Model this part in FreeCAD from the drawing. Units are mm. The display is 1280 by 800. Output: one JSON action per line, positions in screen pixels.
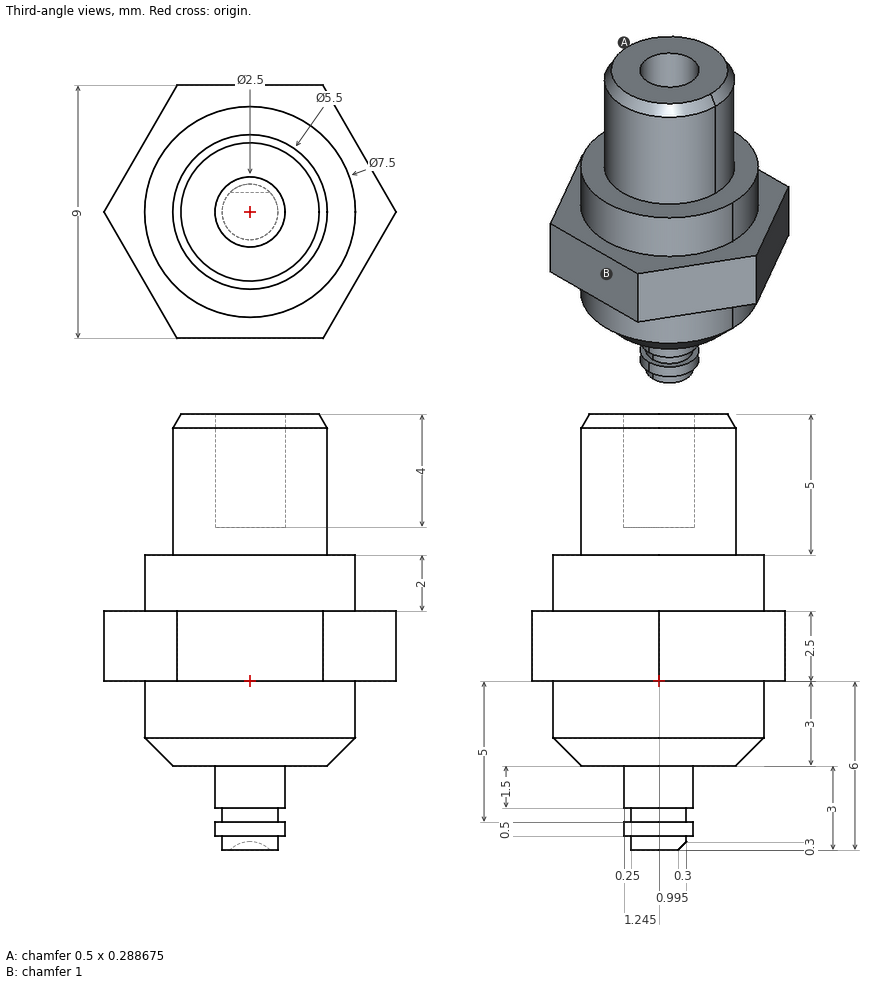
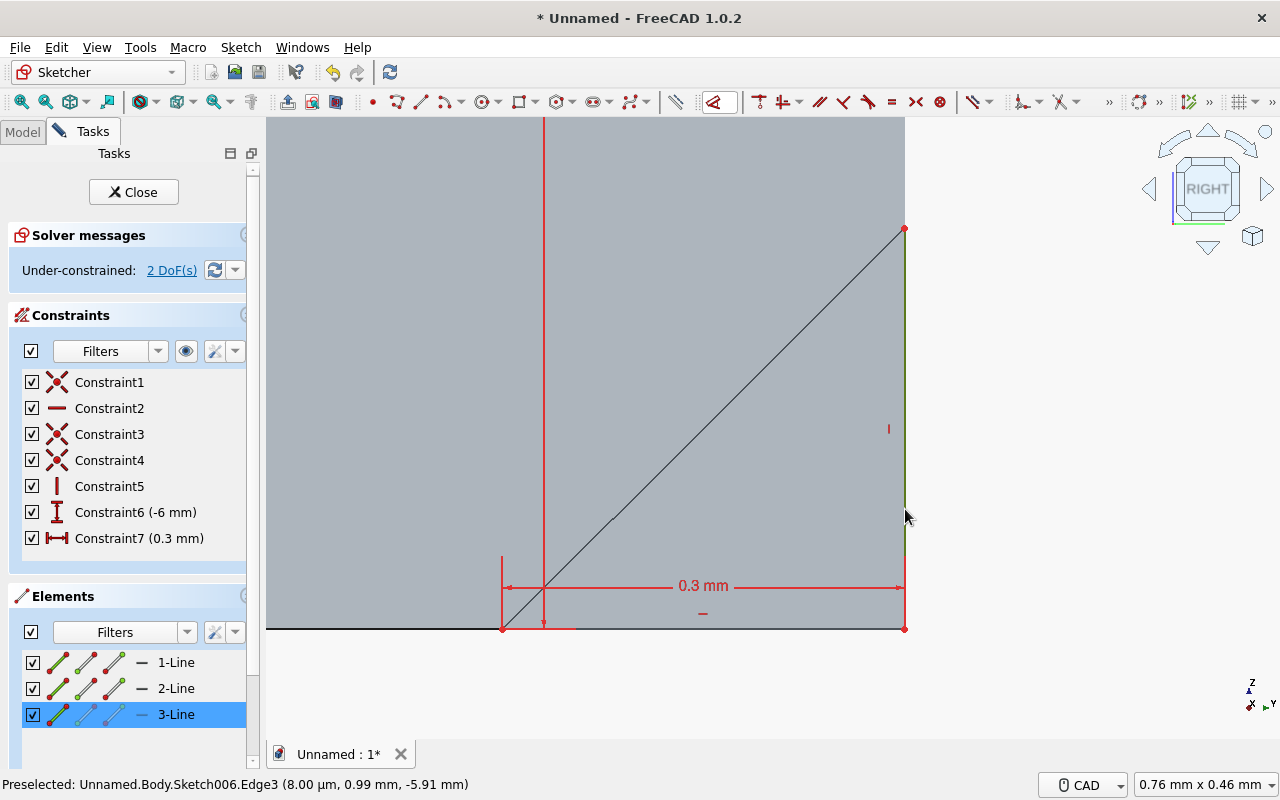
{"action": "key", "text": "i"}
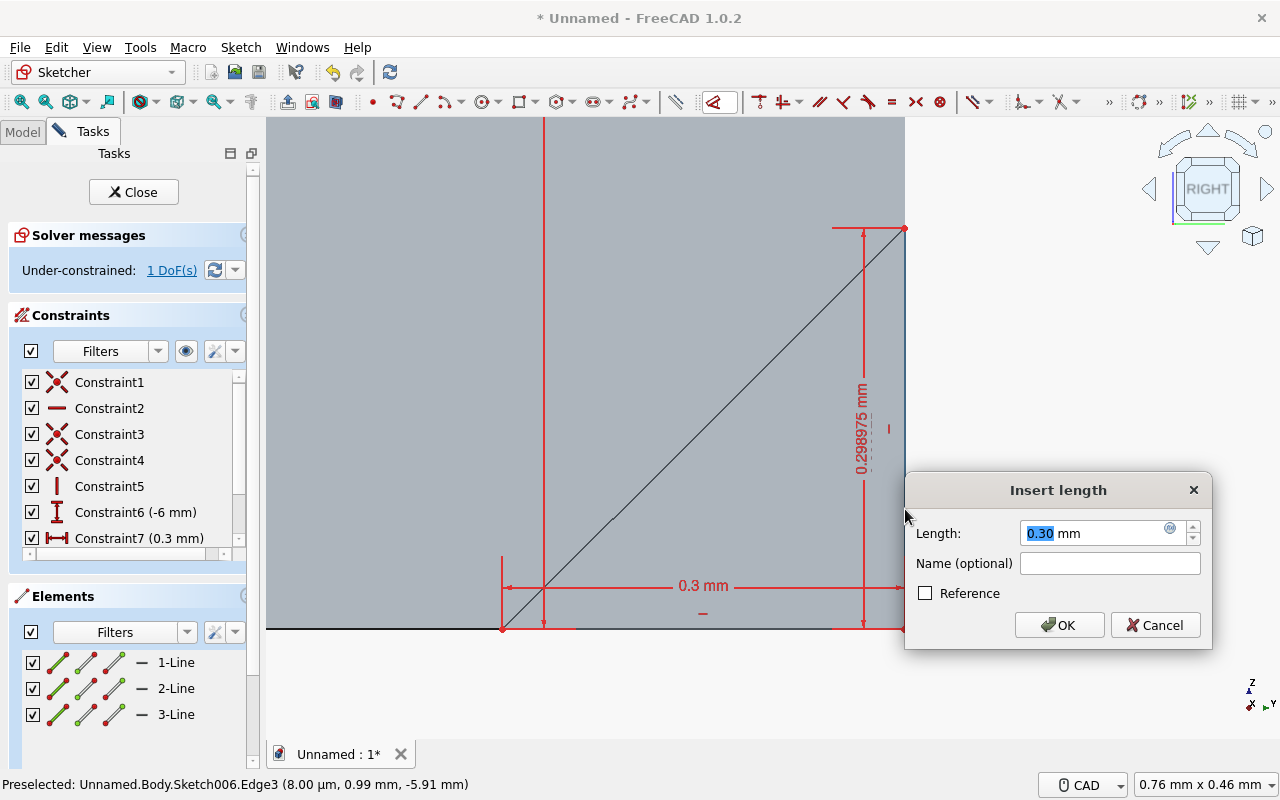
{"action": "type", "text": "0.3"}
{"action": "key", "text": "Return"}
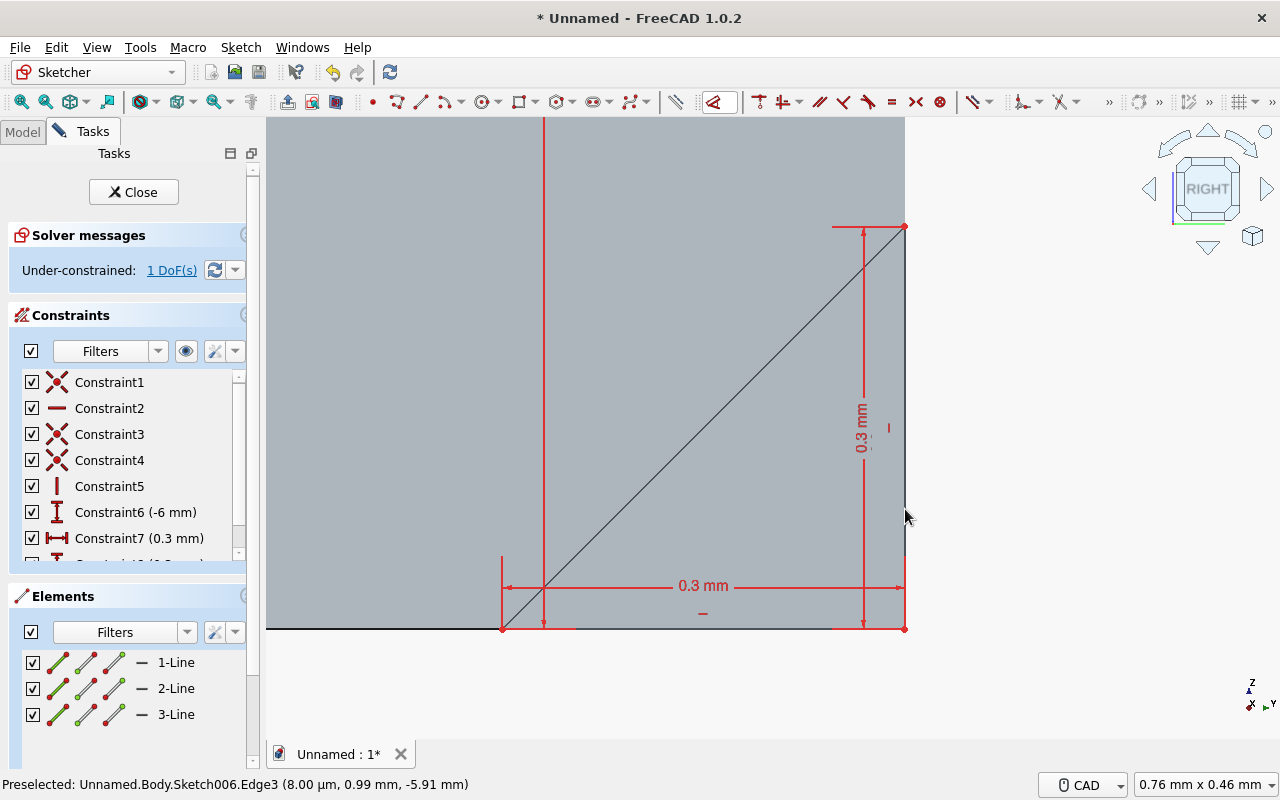
{"action": "left_click", "coordinate": [905, 227]}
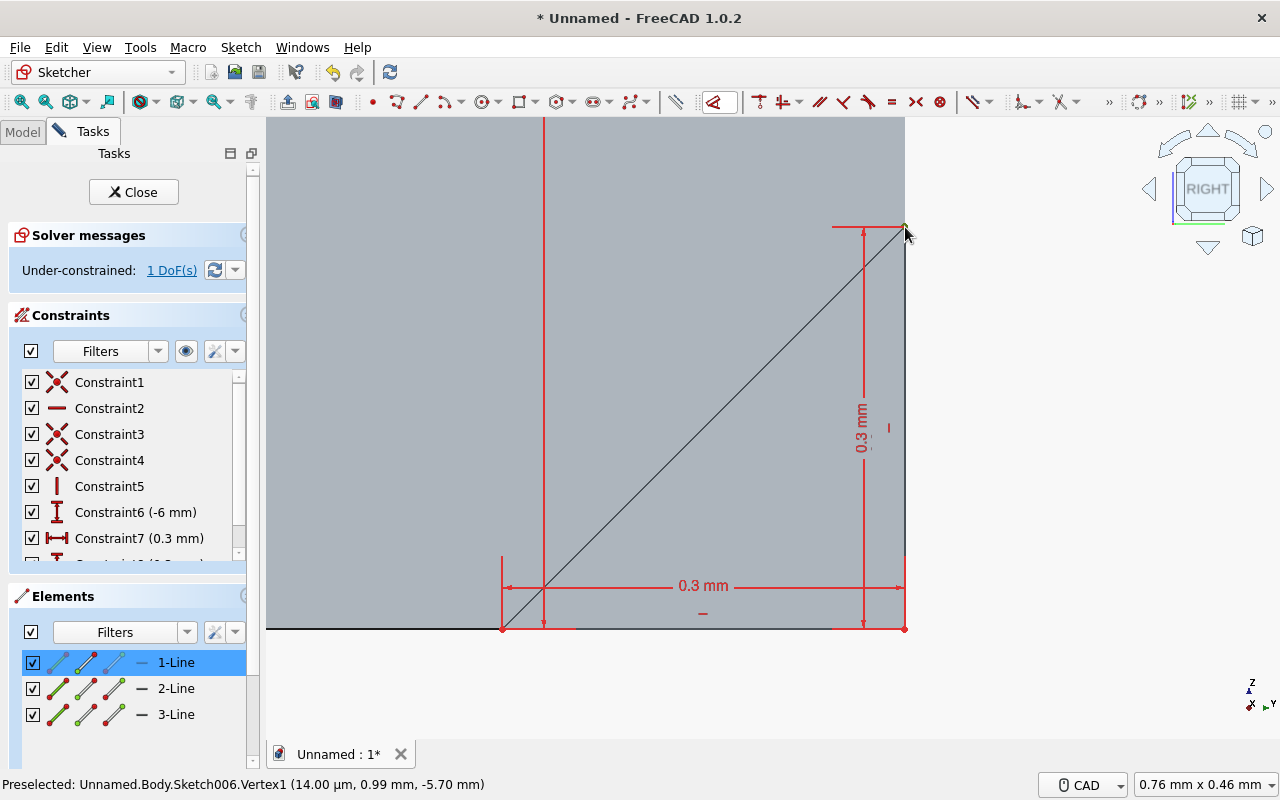
{"action": "key", "text": "l"}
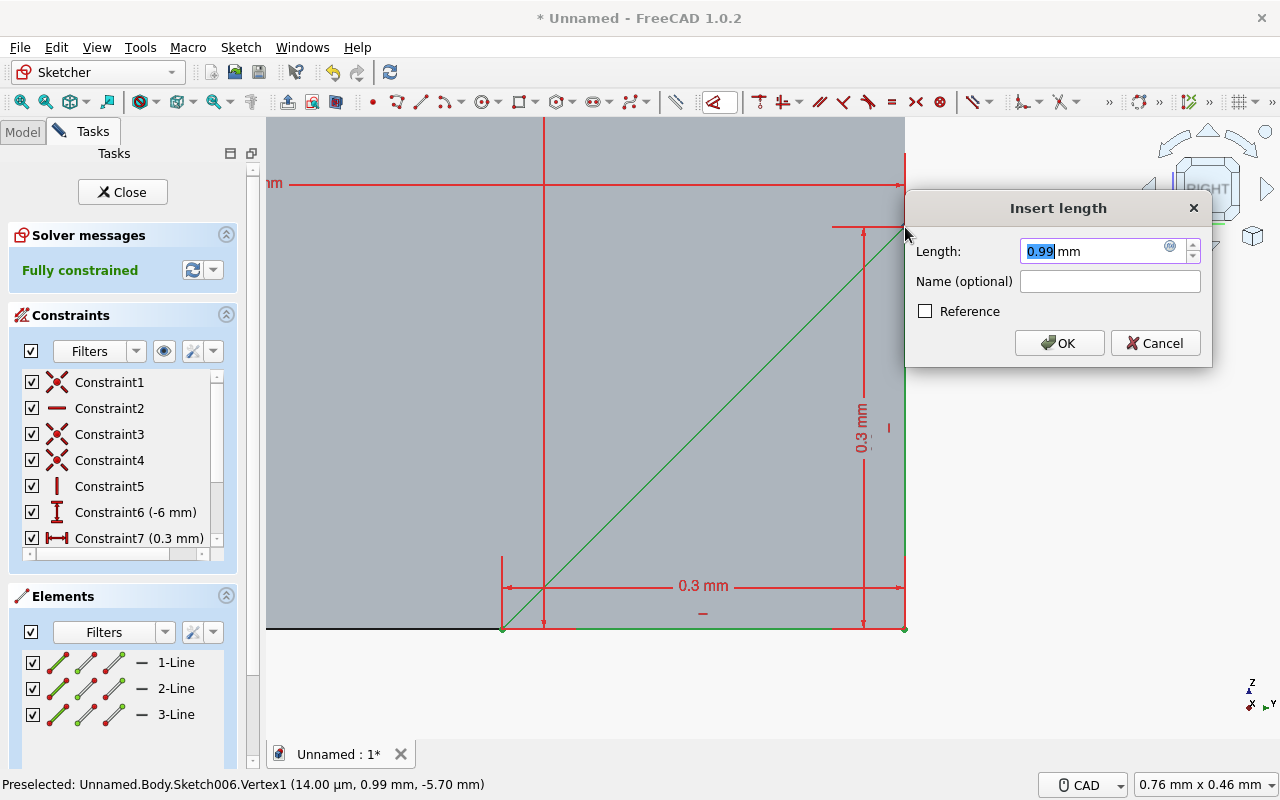
{"action": "type", "text": "0.995"}
{"action": "key", "text": "Return"}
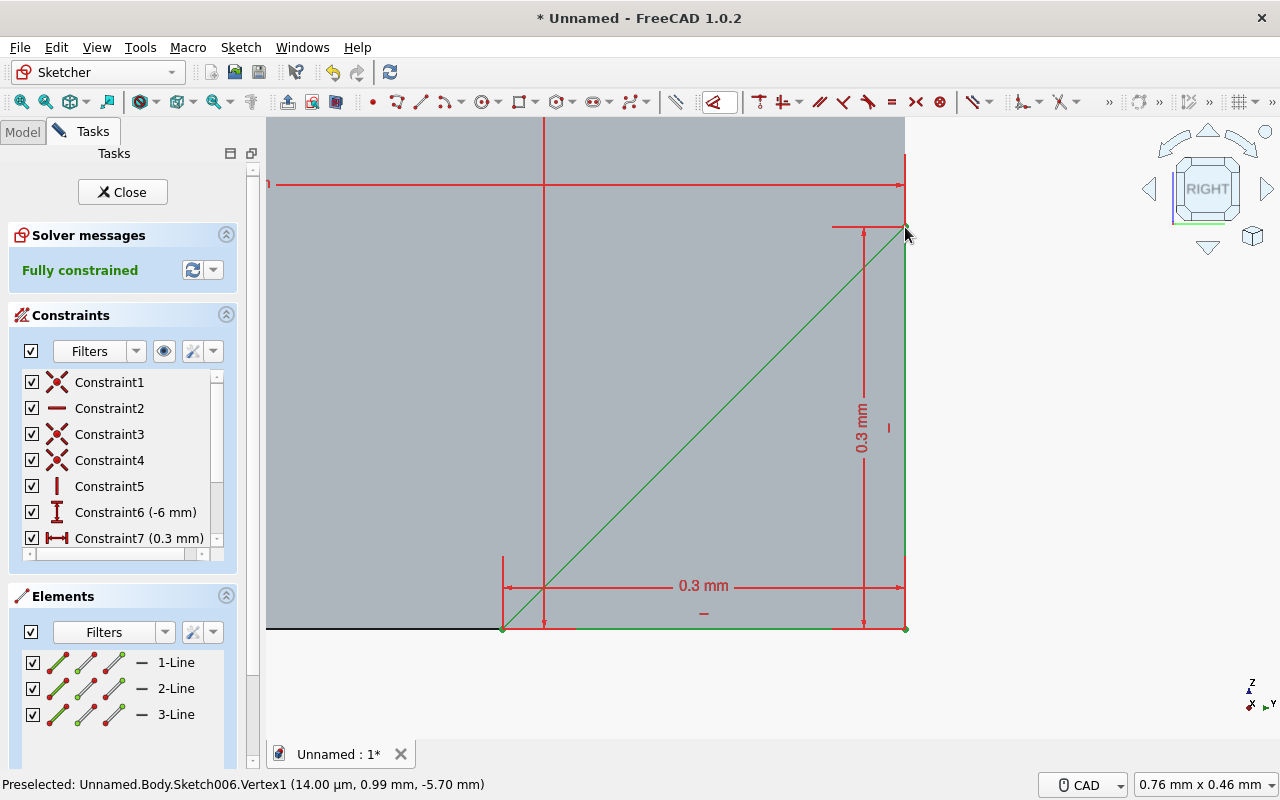
{"action": "left_click", "coordinate": [123, 192]}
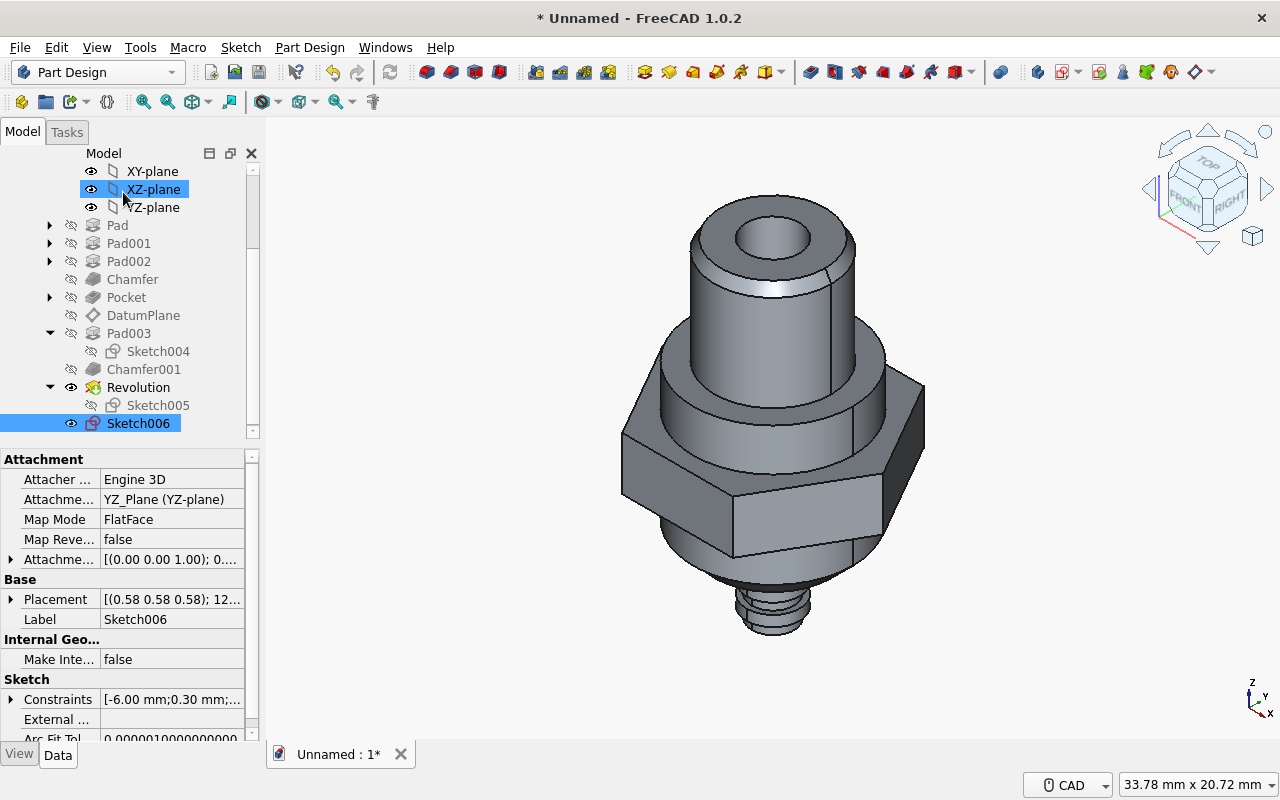
{"action": "left_click", "coordinate": [812, 72]}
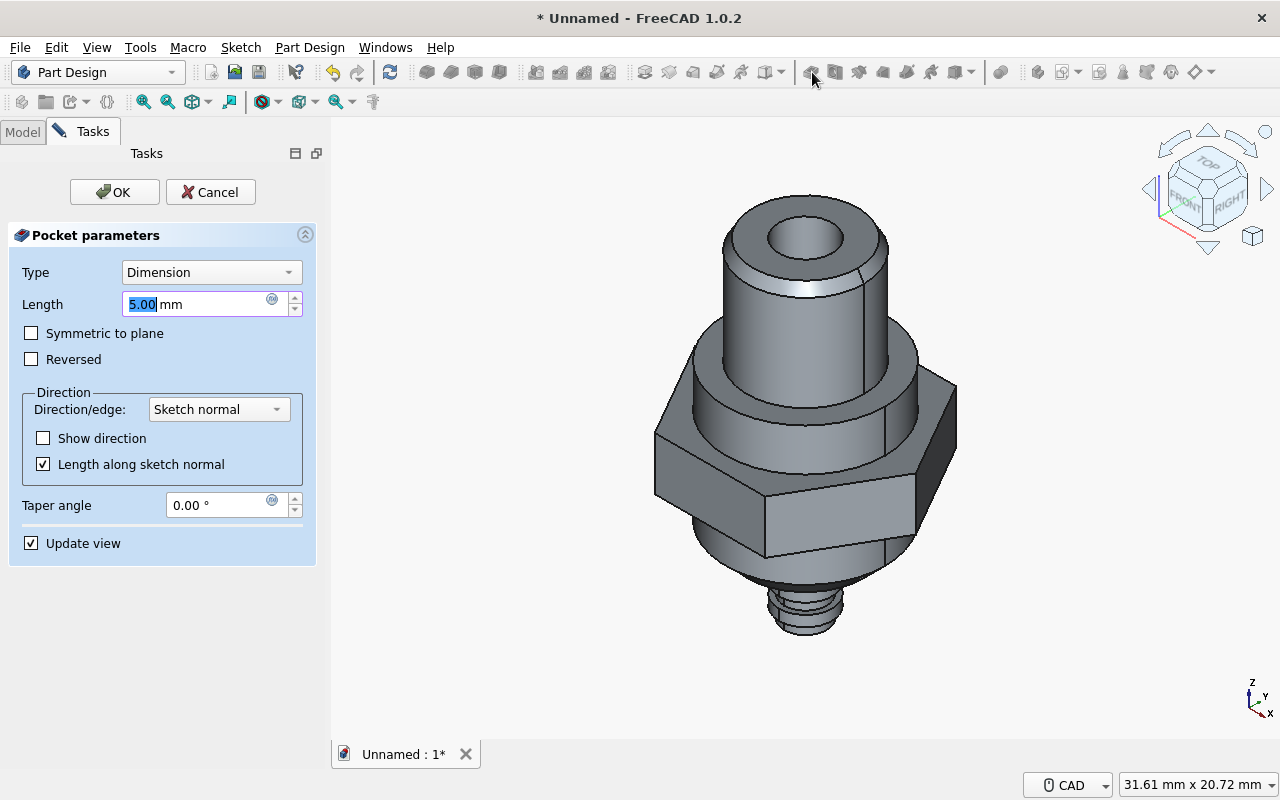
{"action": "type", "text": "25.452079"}
{"action": "key", "text": "Tab"}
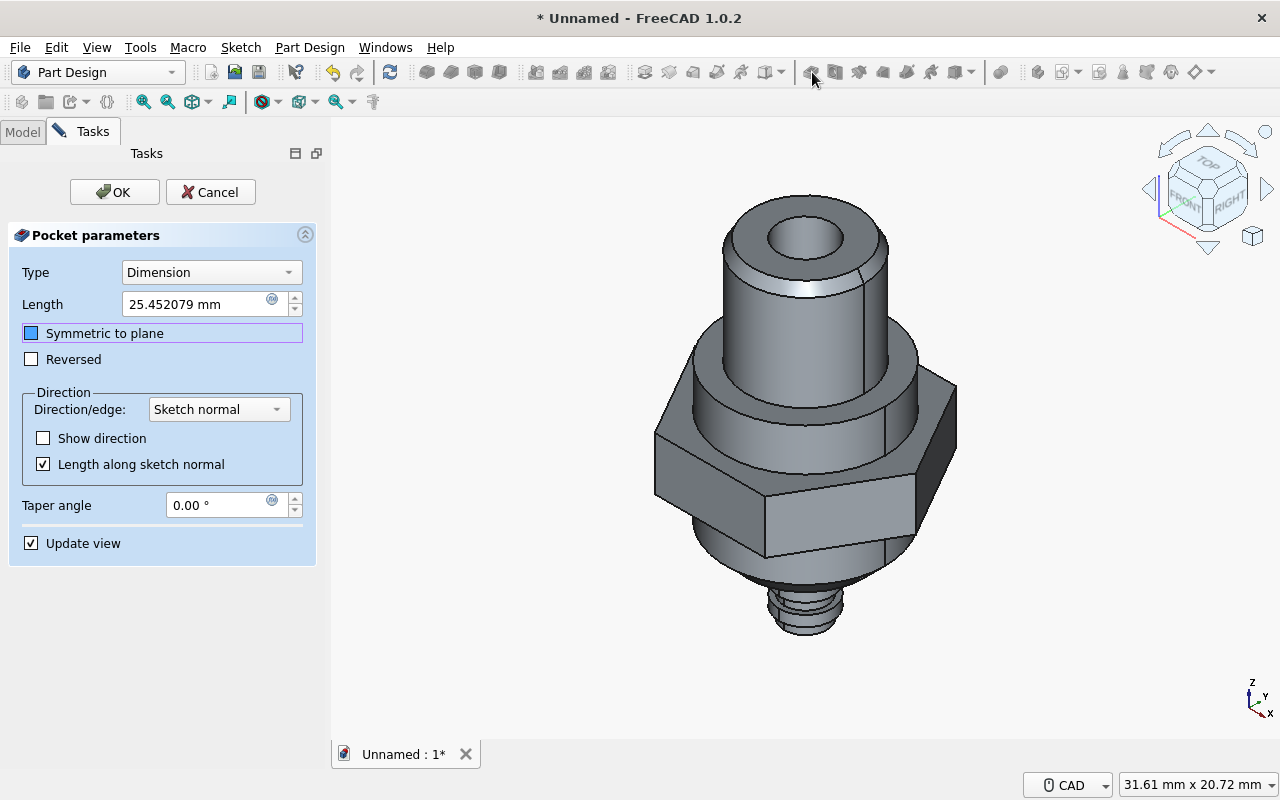
{"action": "left_click", "coordinate": [30, 333]}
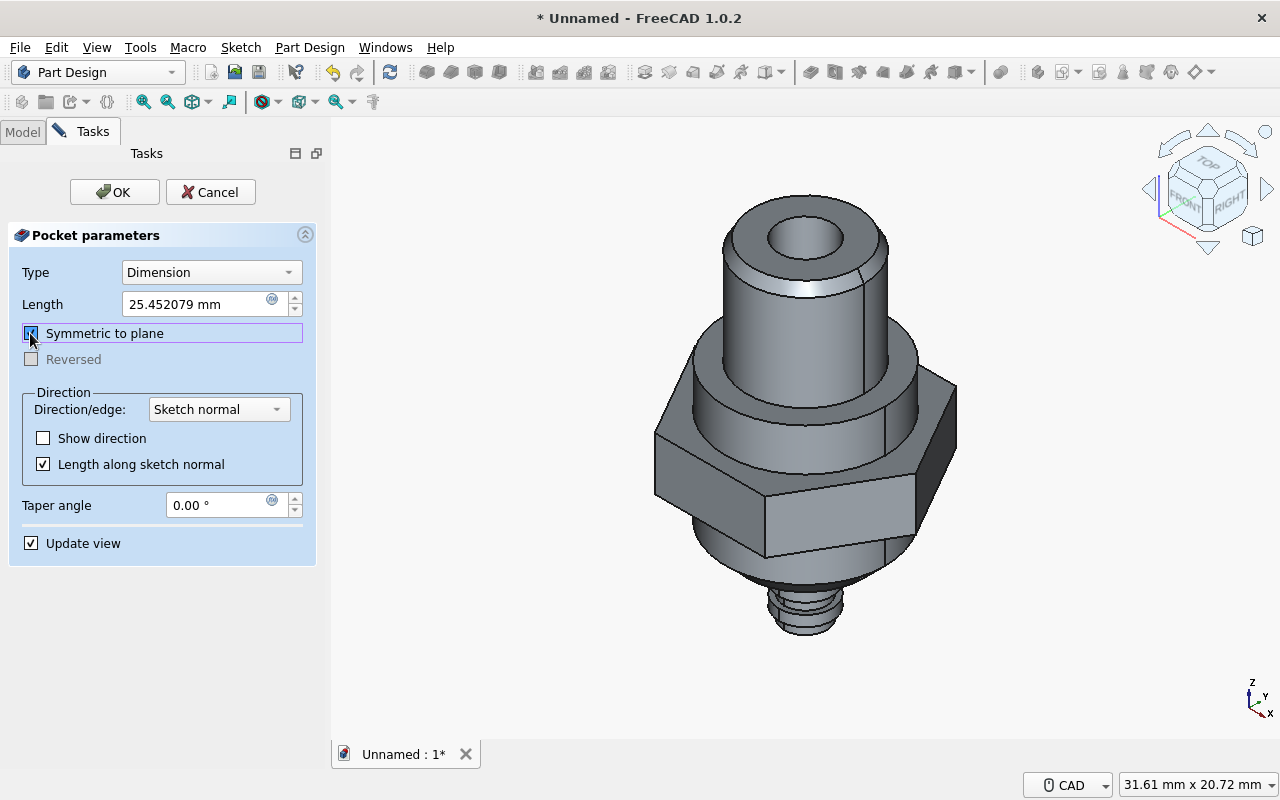
{"action": "left_click", "coordinate": [115, 192]}